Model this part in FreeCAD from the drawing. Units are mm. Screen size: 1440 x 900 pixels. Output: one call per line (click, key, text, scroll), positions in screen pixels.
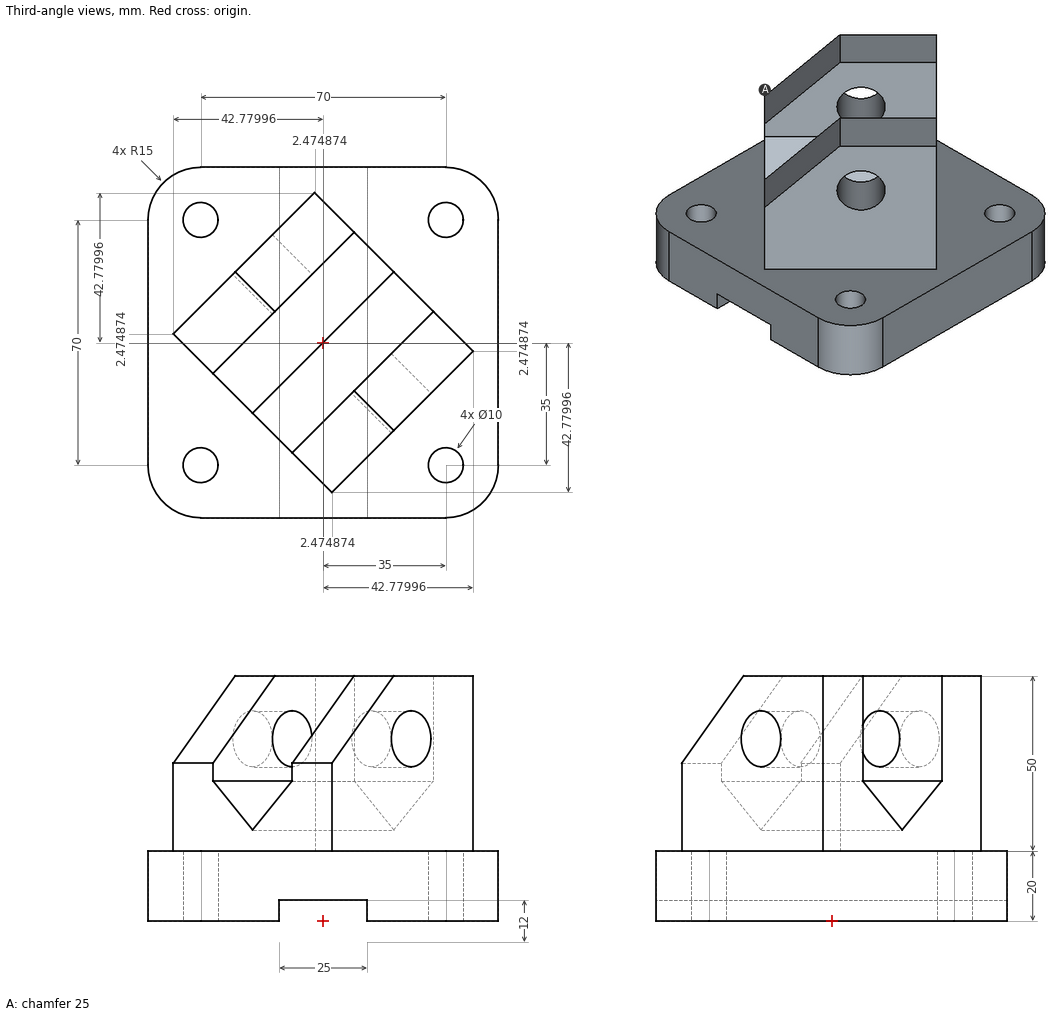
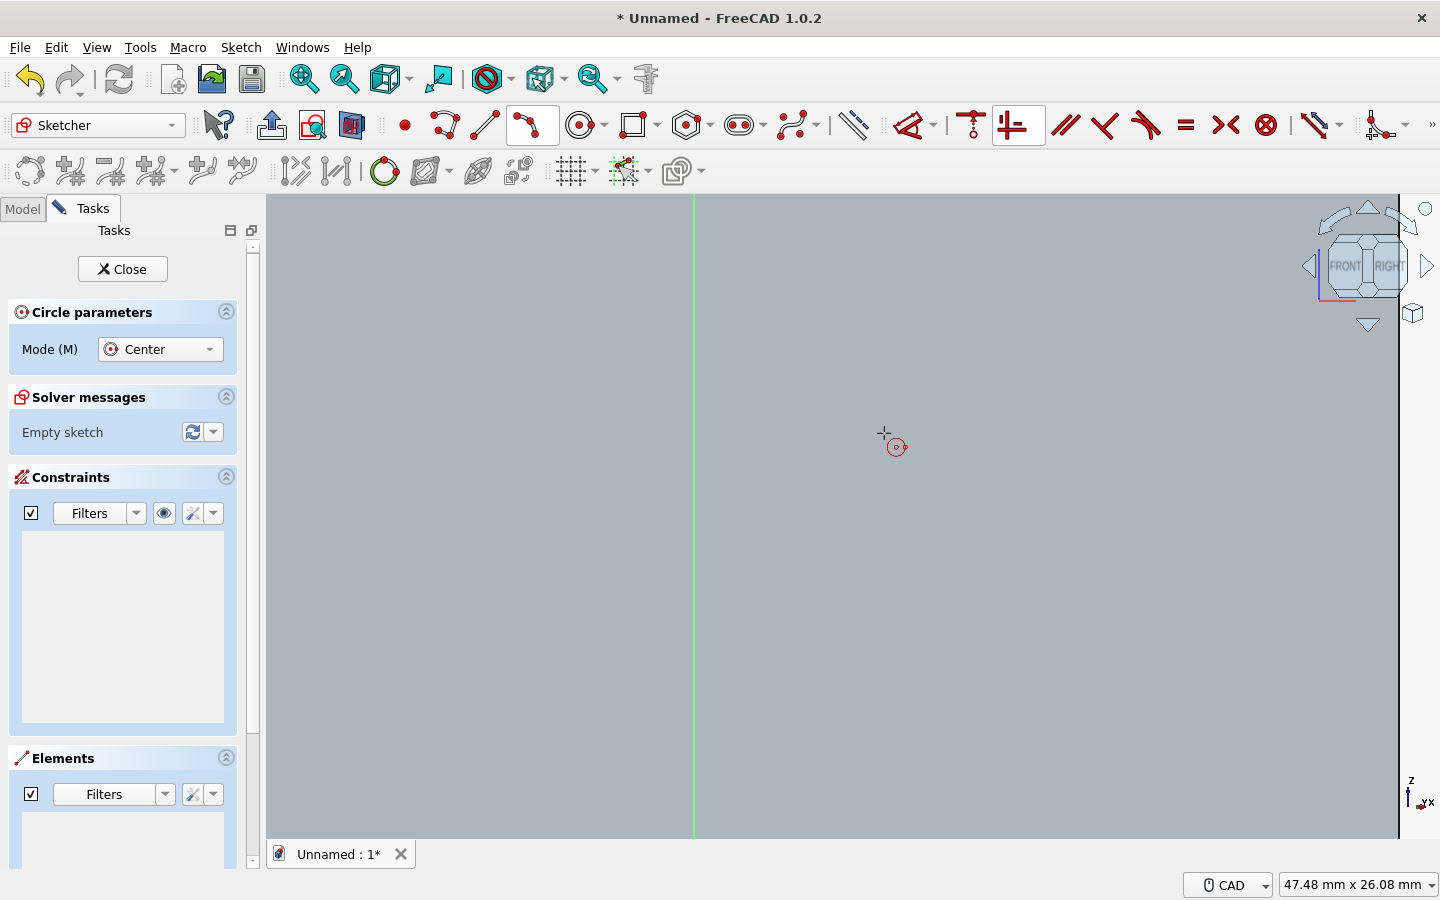
click(780, 516)
move(920, 376)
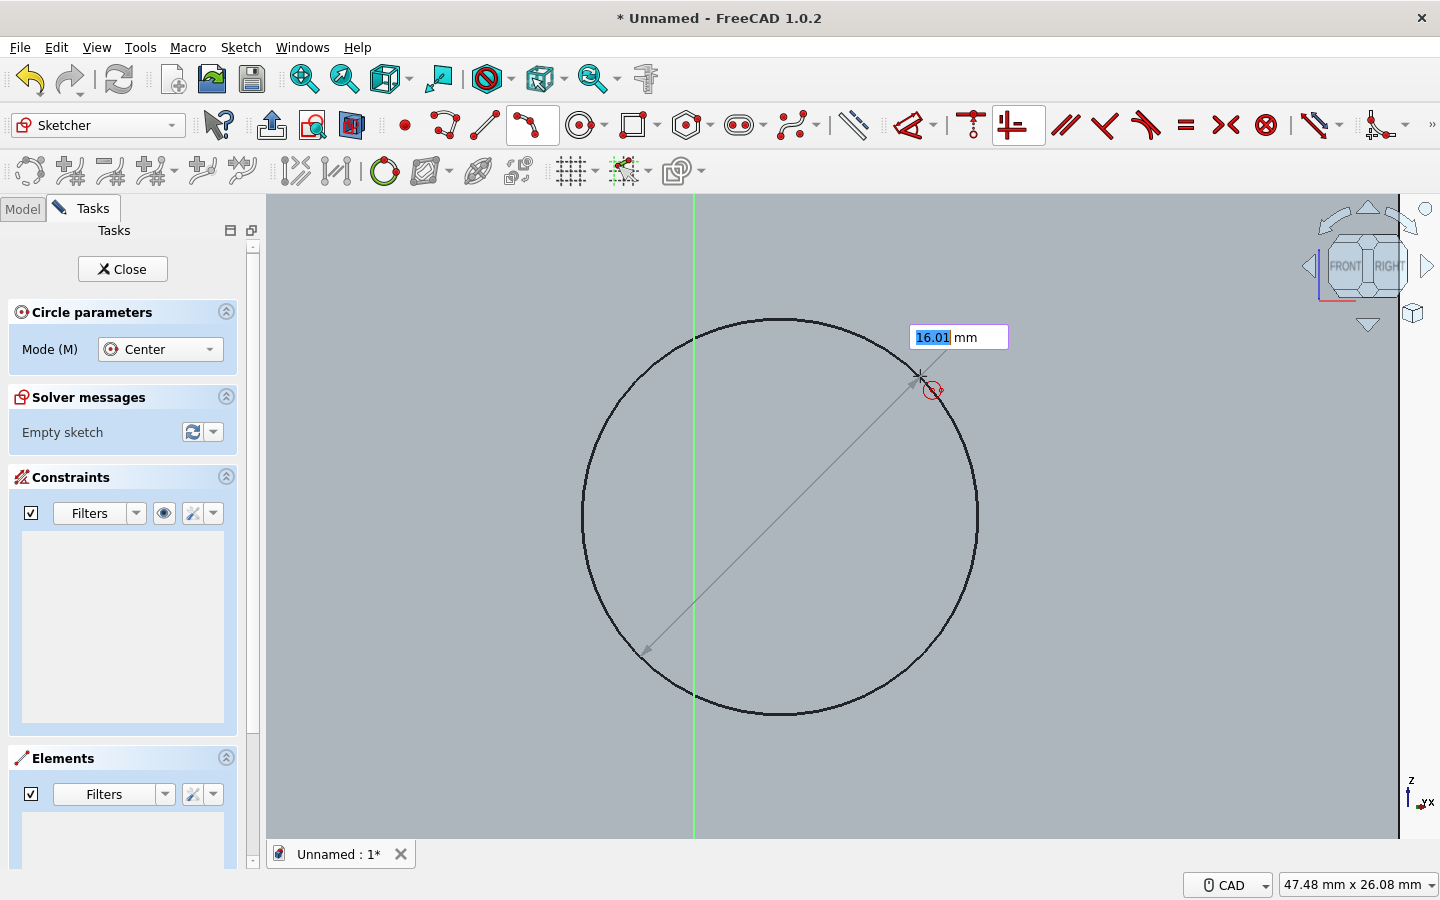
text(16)
key(Return)
key(Escape)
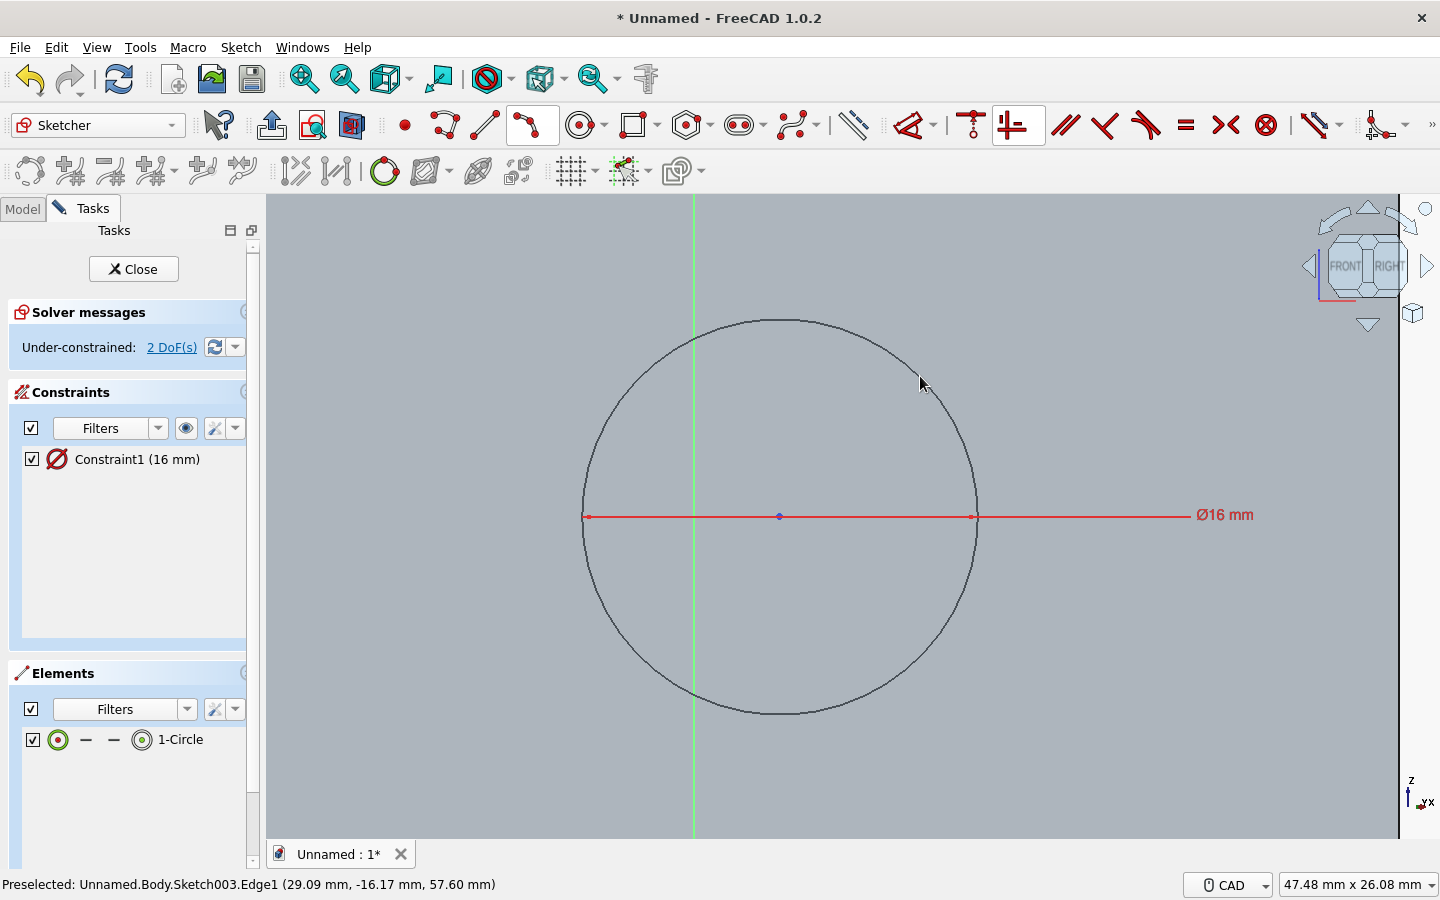
click(908, 126)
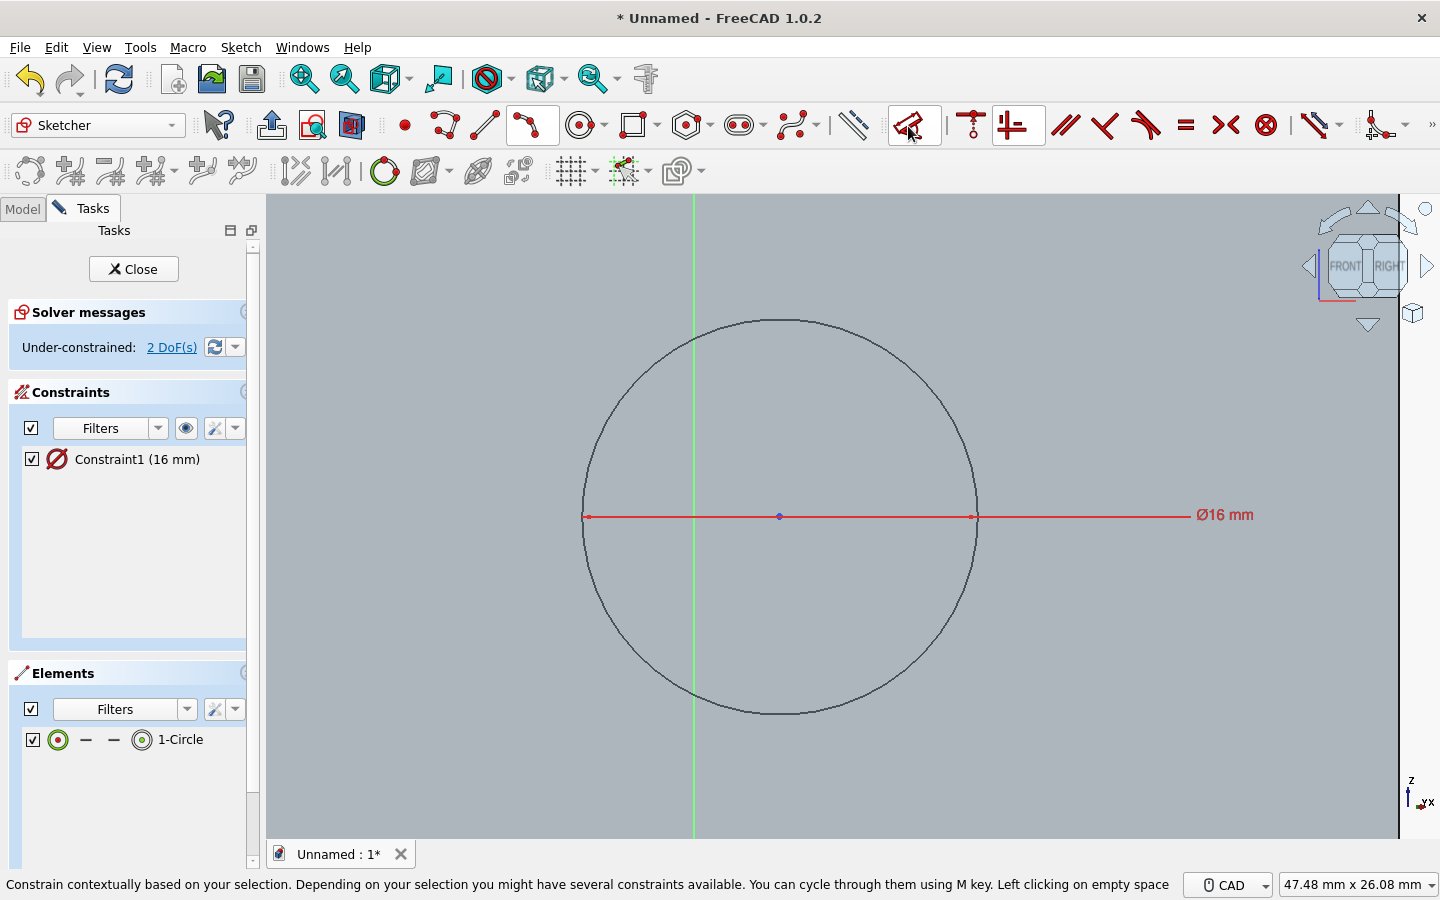
click(780, 517)
click(660, 596)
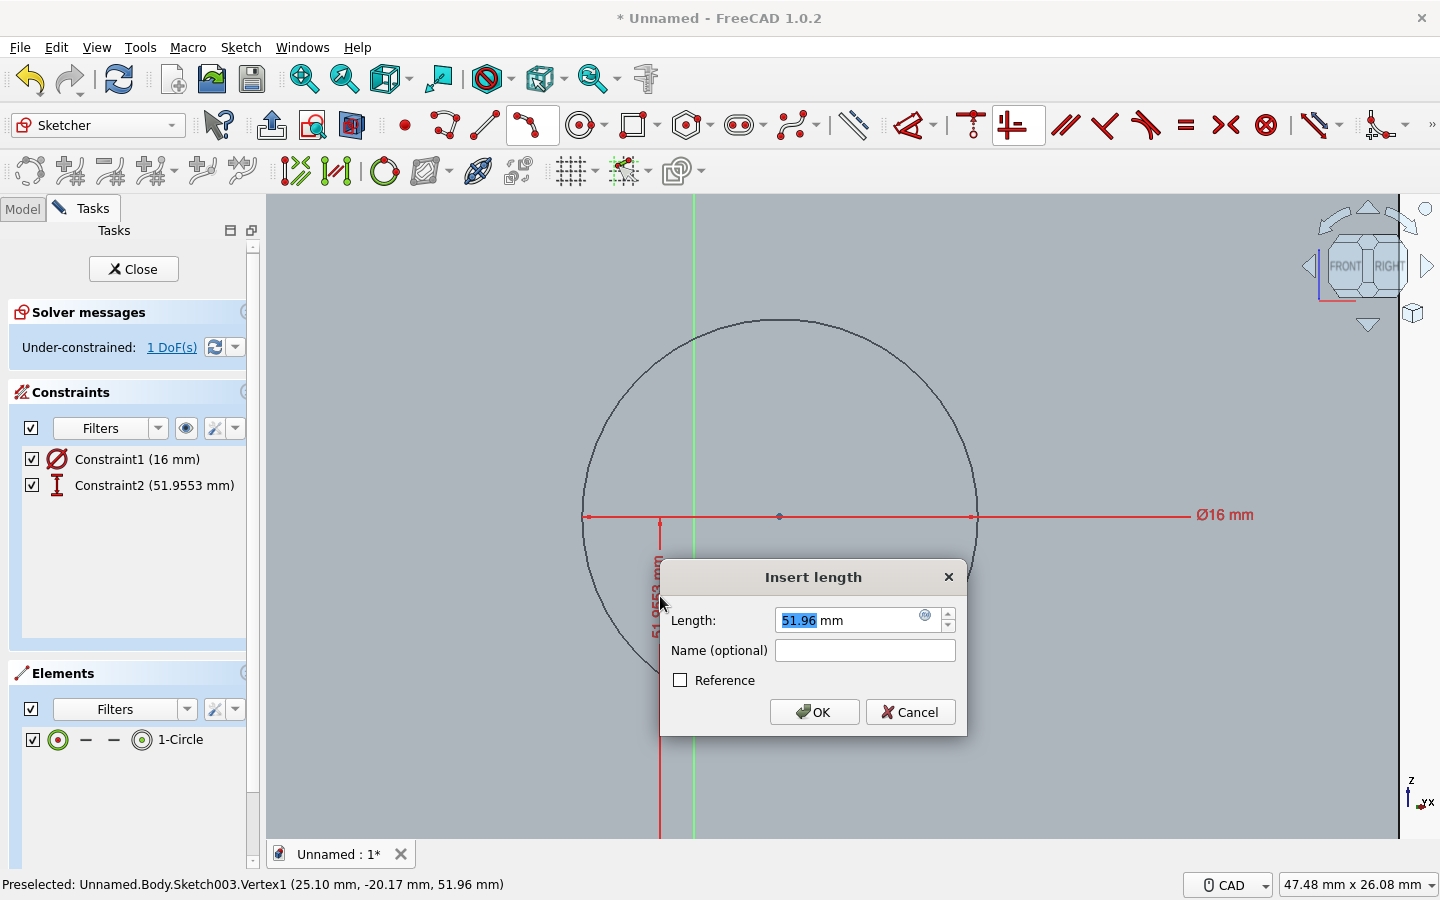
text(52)
key(Return)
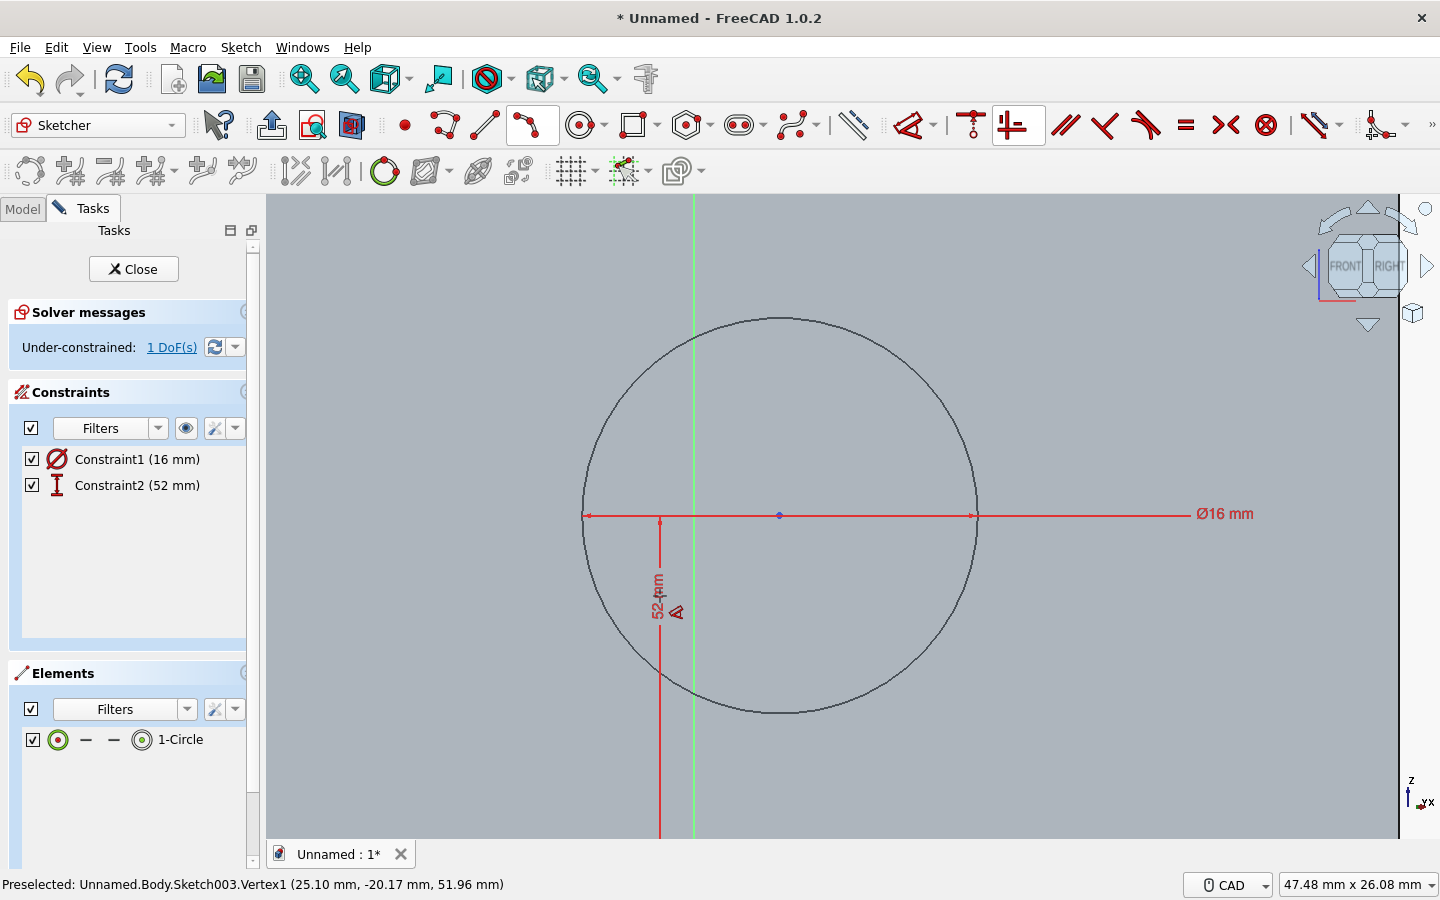
click(780, 516)
click(737, 482)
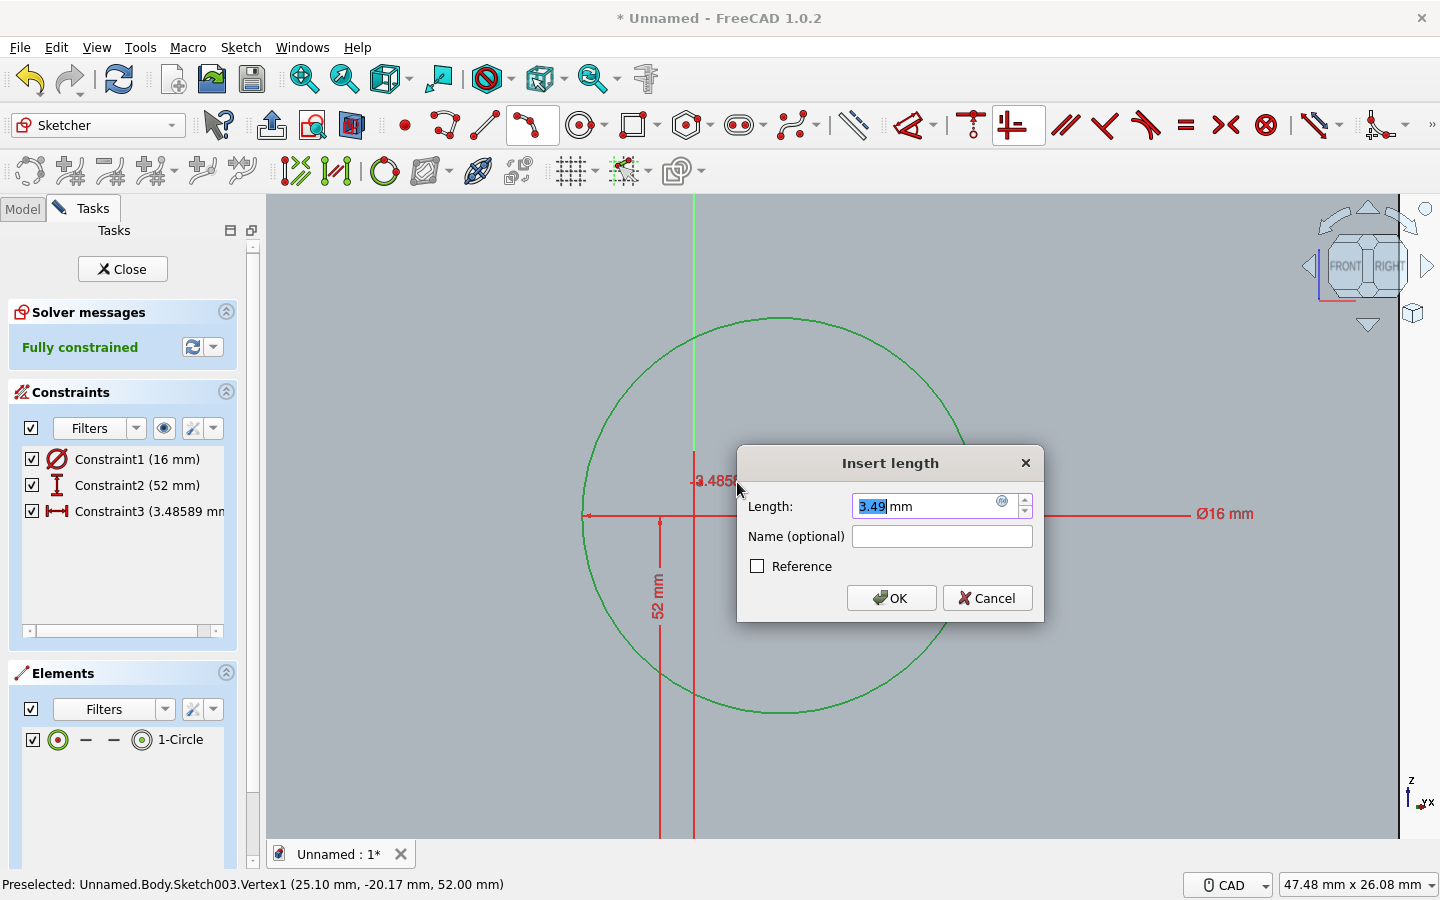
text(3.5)
key(Return)
key(Escape)